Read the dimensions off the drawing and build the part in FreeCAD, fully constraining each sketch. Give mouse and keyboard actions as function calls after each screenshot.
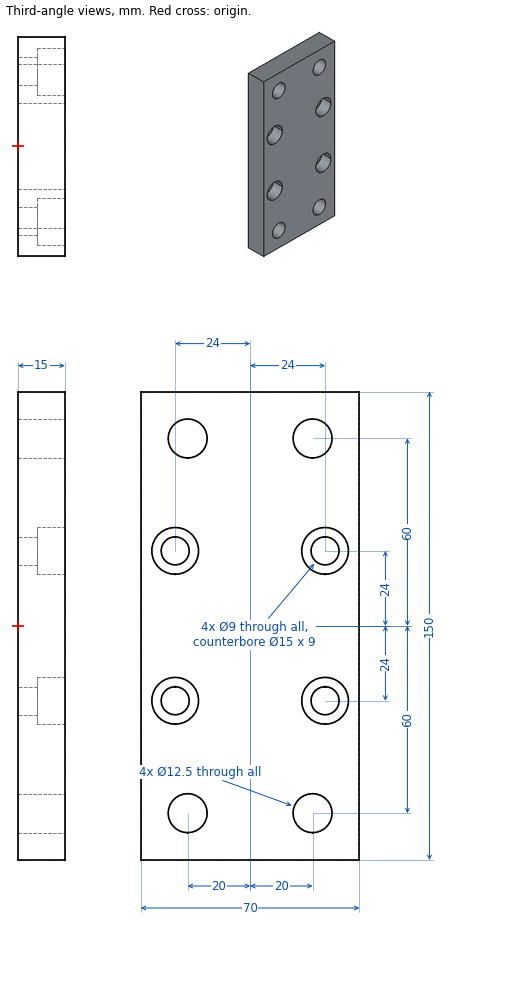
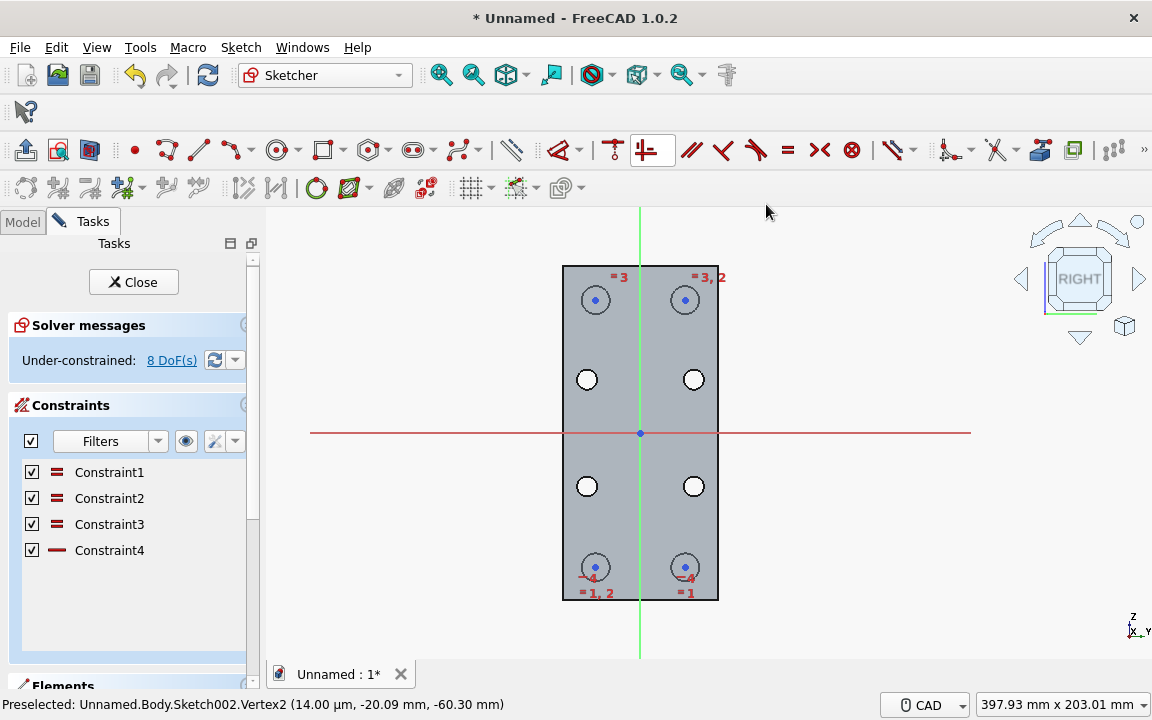
click(685, 567)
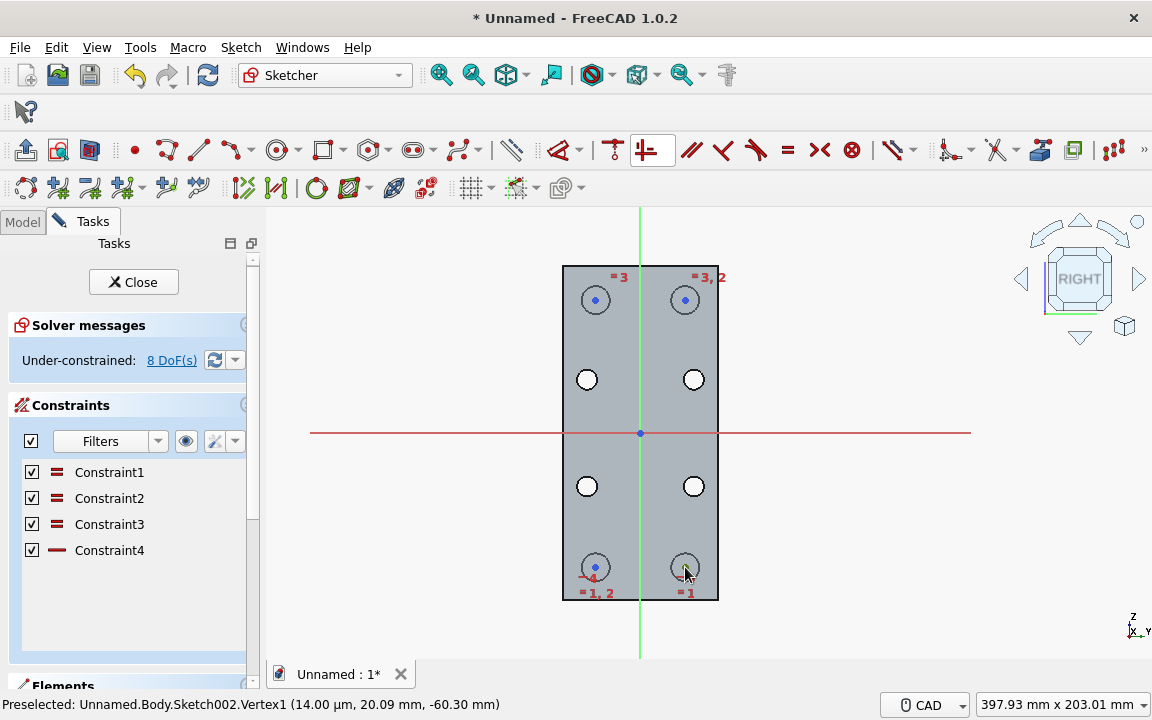
click(685, 300)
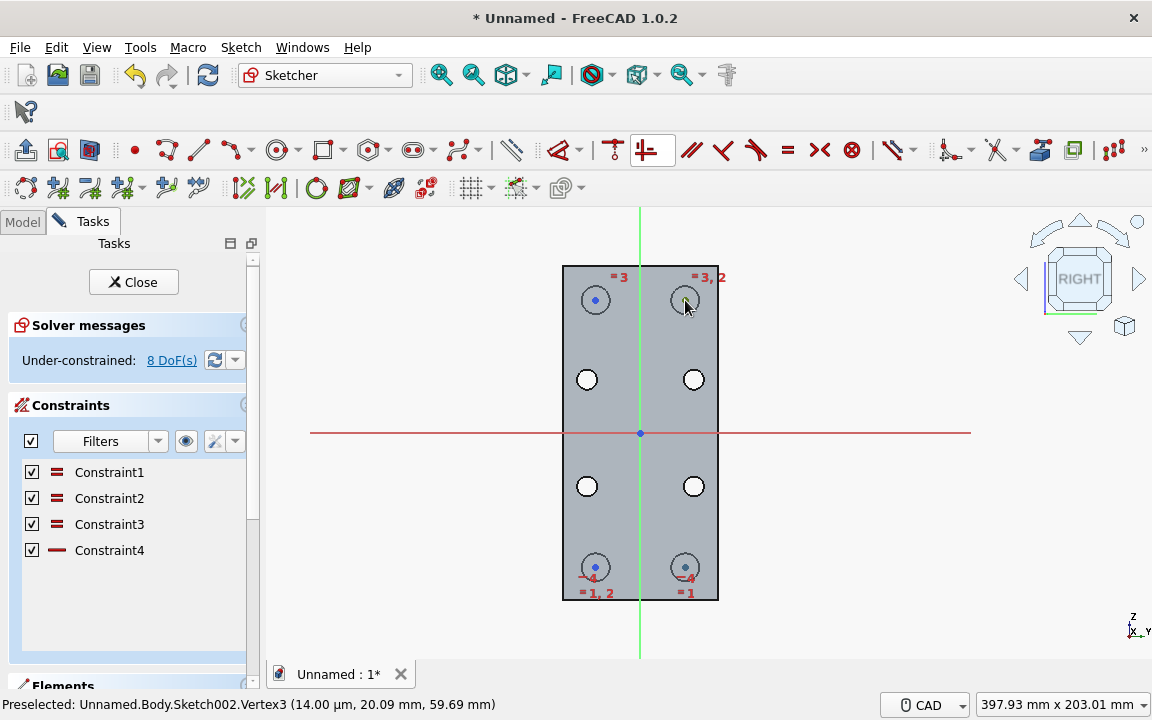
key(v)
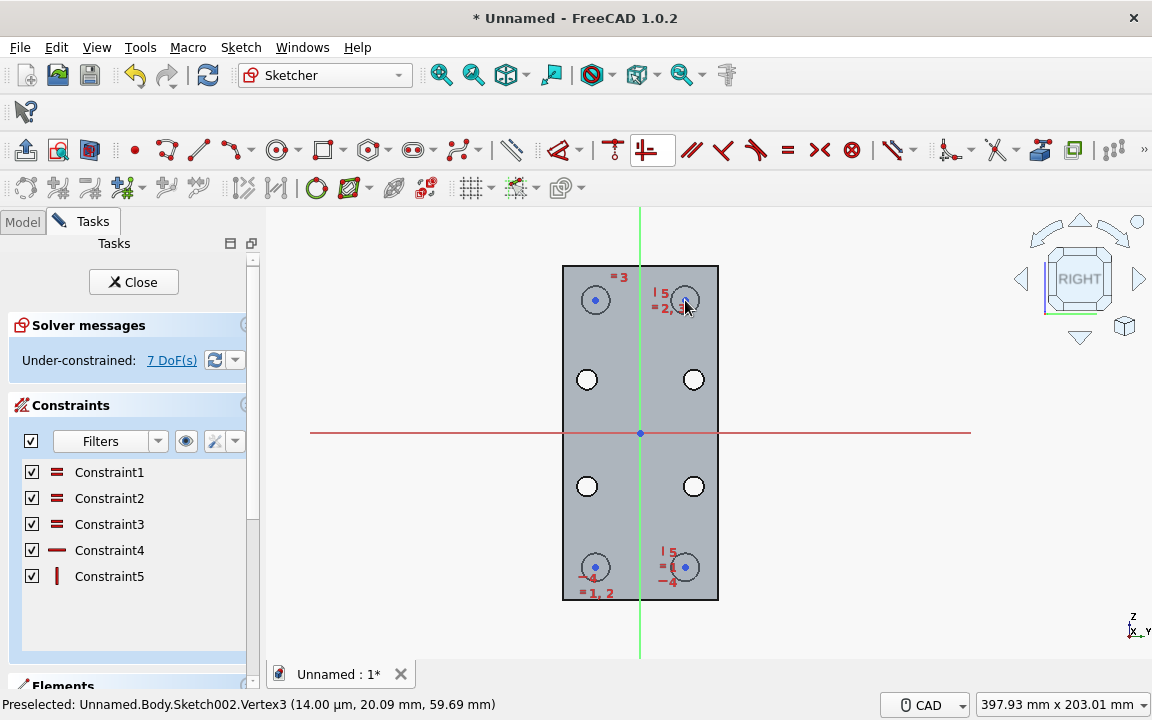
click(596, 567)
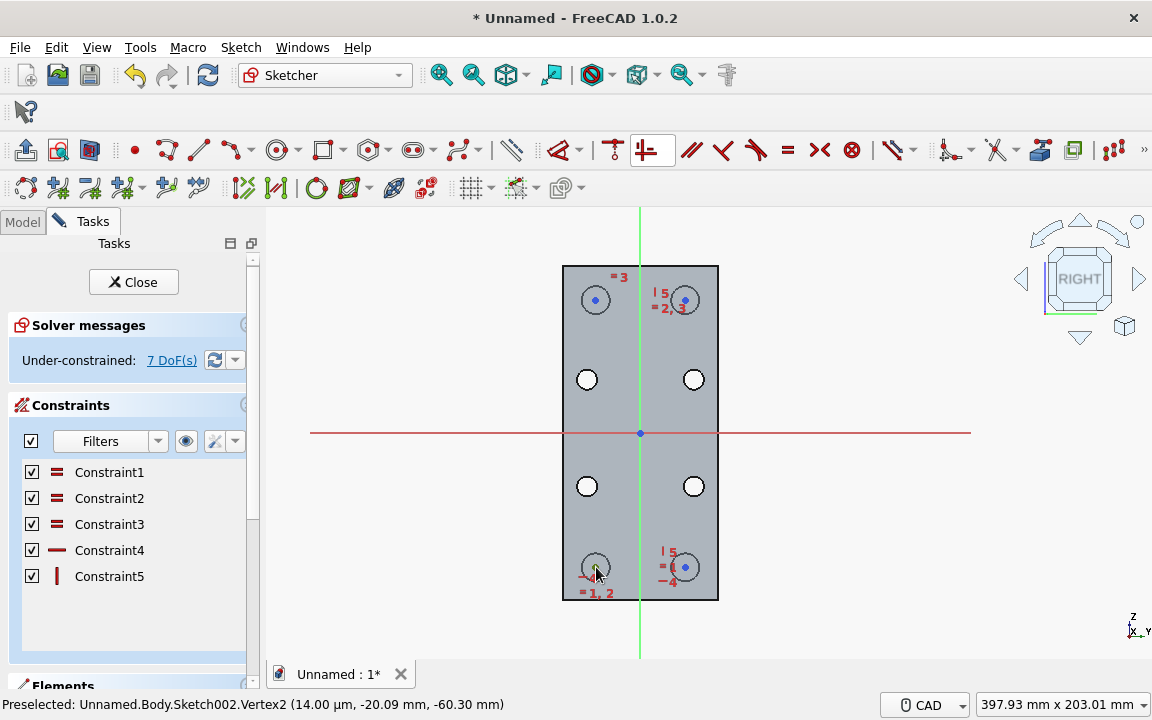
click(596, 300)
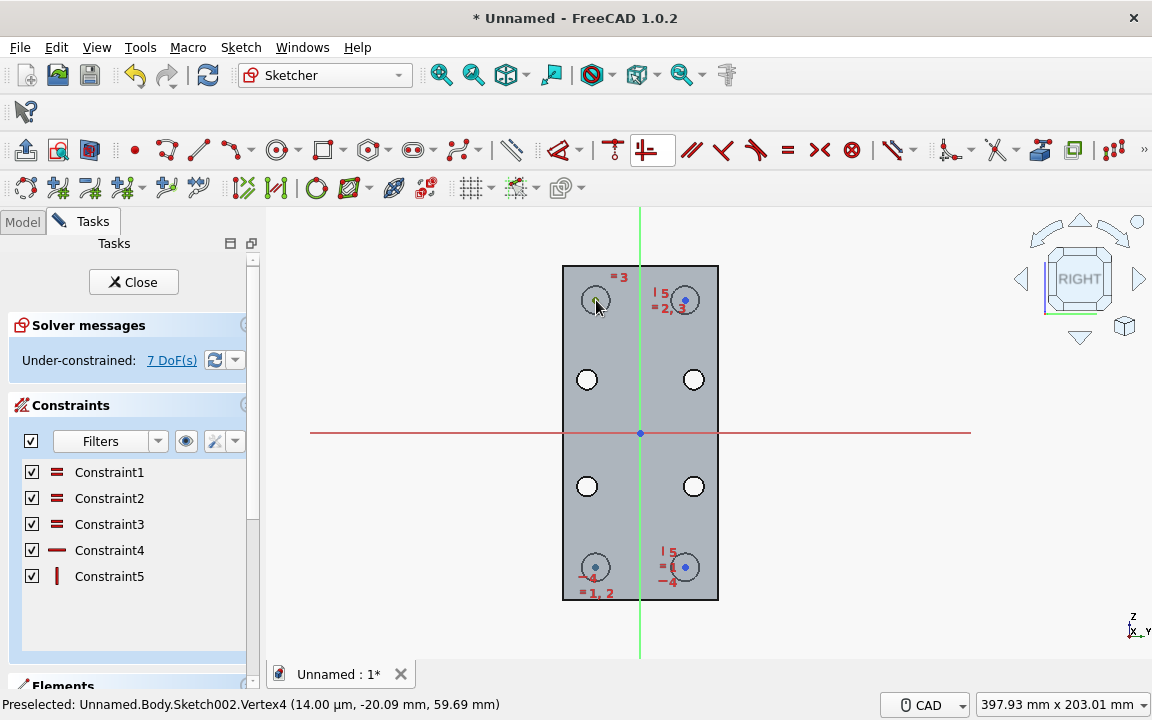
click(670, 150)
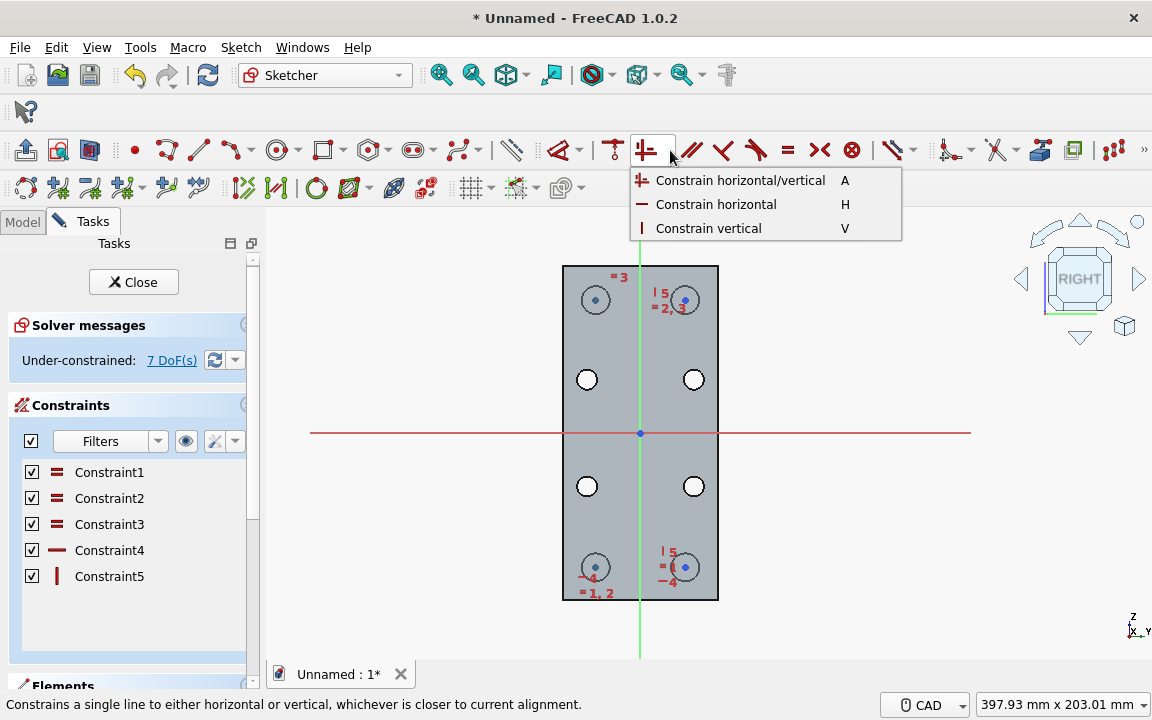
click(766, 228)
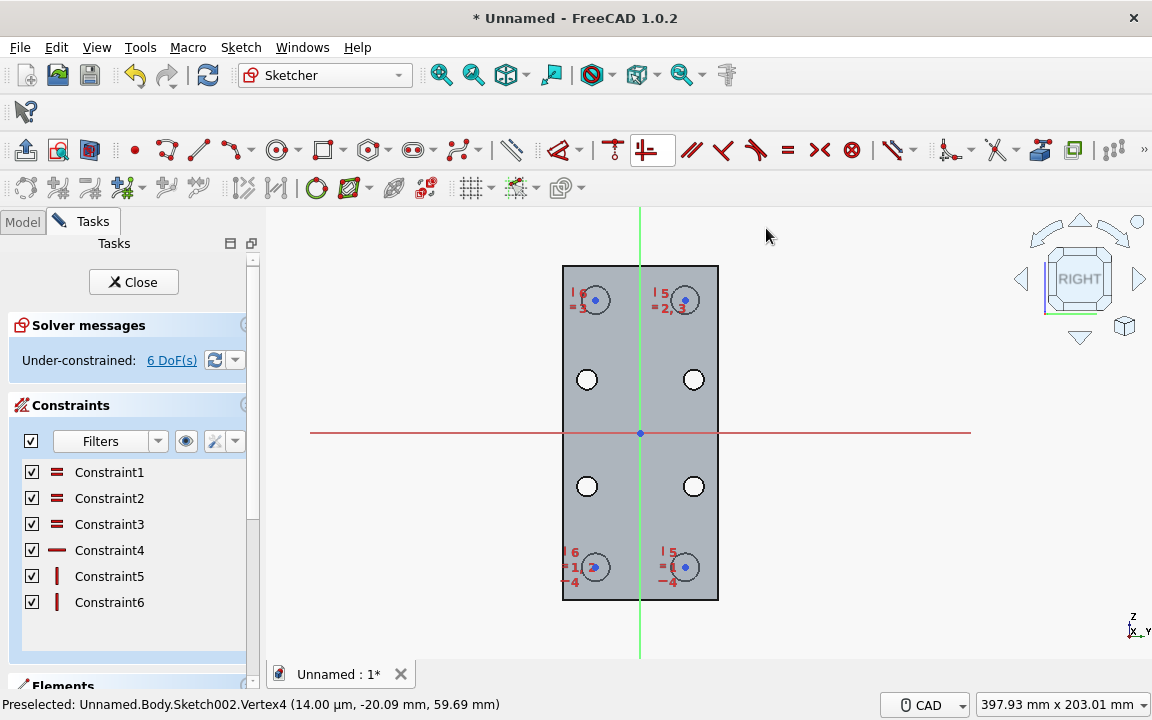
click(687, 302)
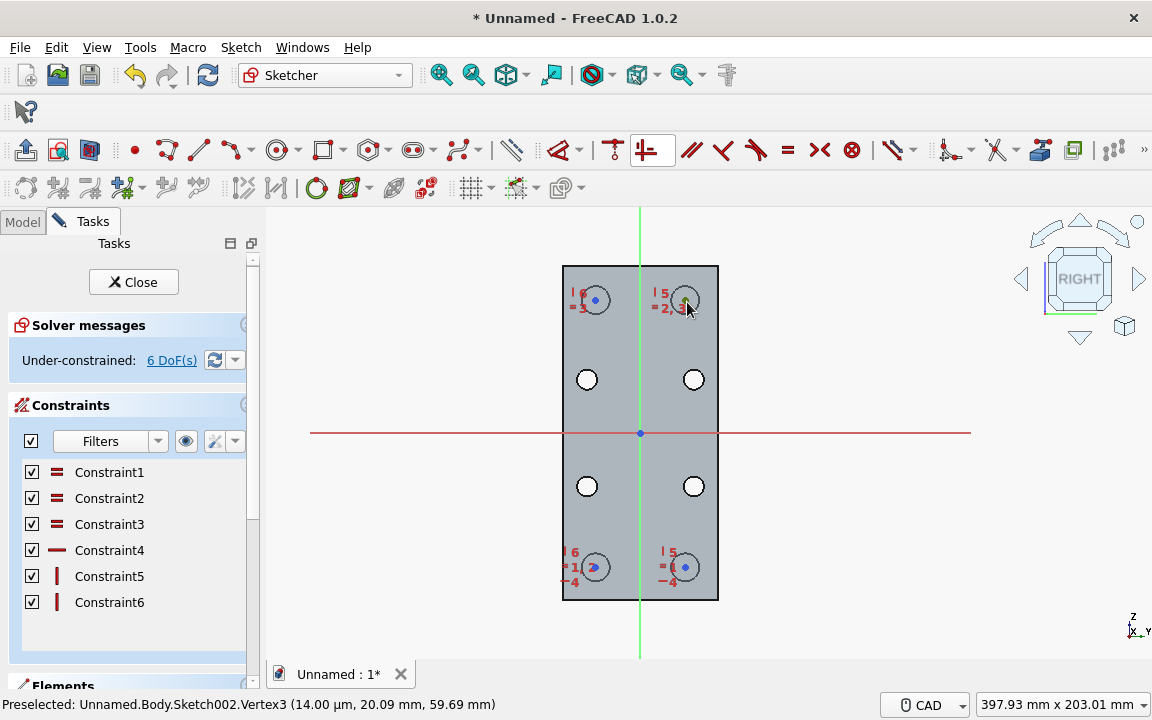
click(596, 300)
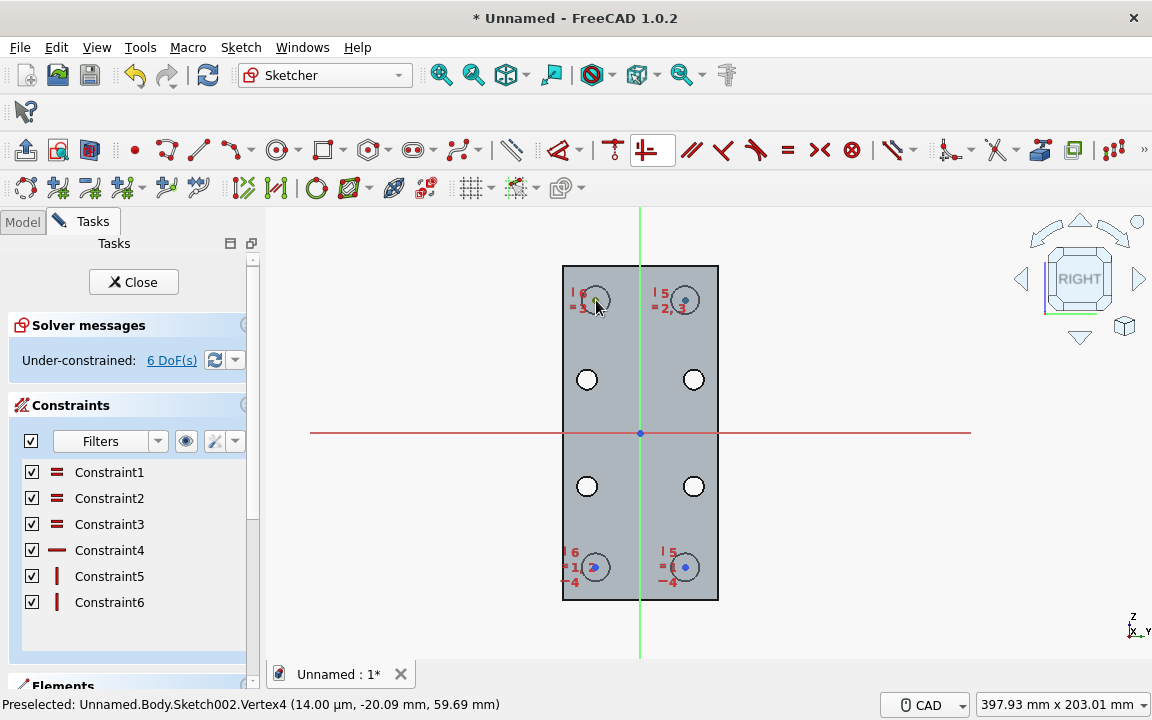
key(h)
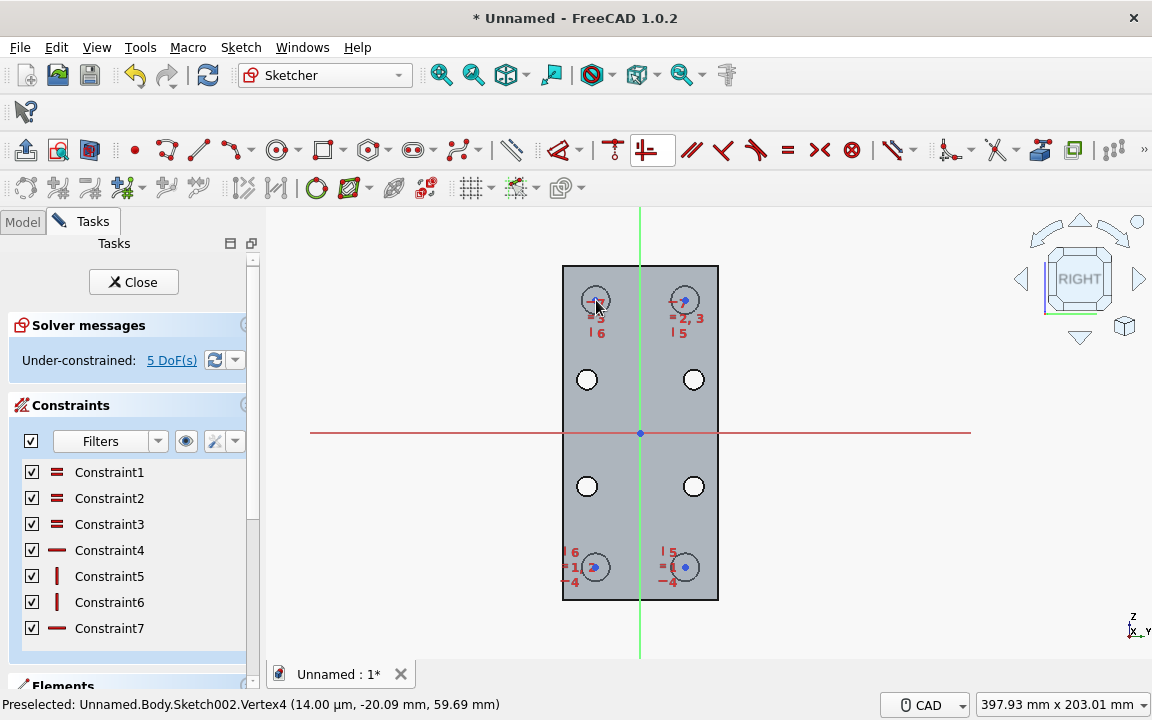
click(558, 150)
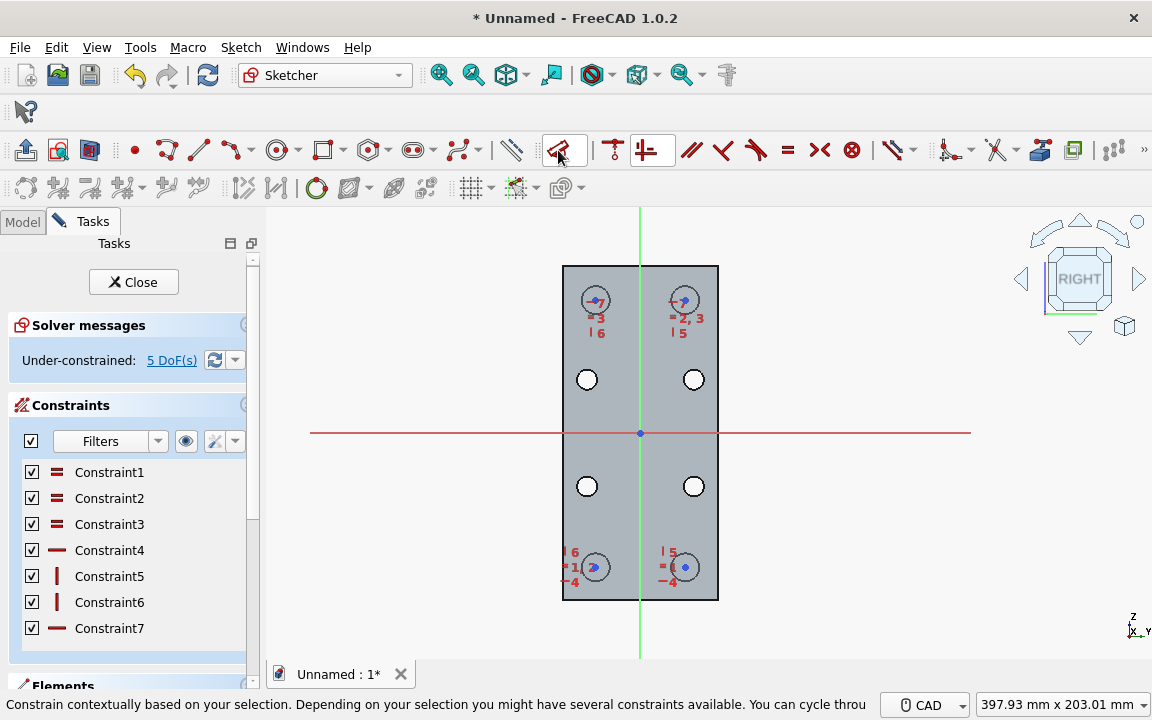
scroll(695, 557, up, 2)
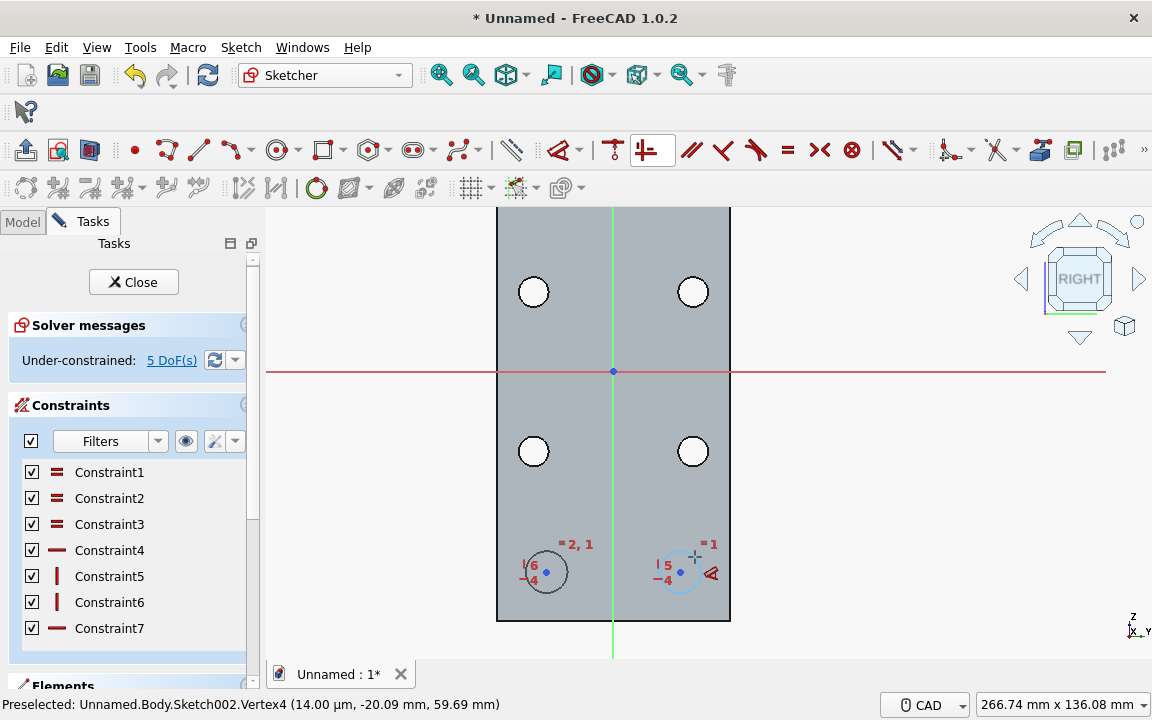
click(695, 557)
click(717, 534)